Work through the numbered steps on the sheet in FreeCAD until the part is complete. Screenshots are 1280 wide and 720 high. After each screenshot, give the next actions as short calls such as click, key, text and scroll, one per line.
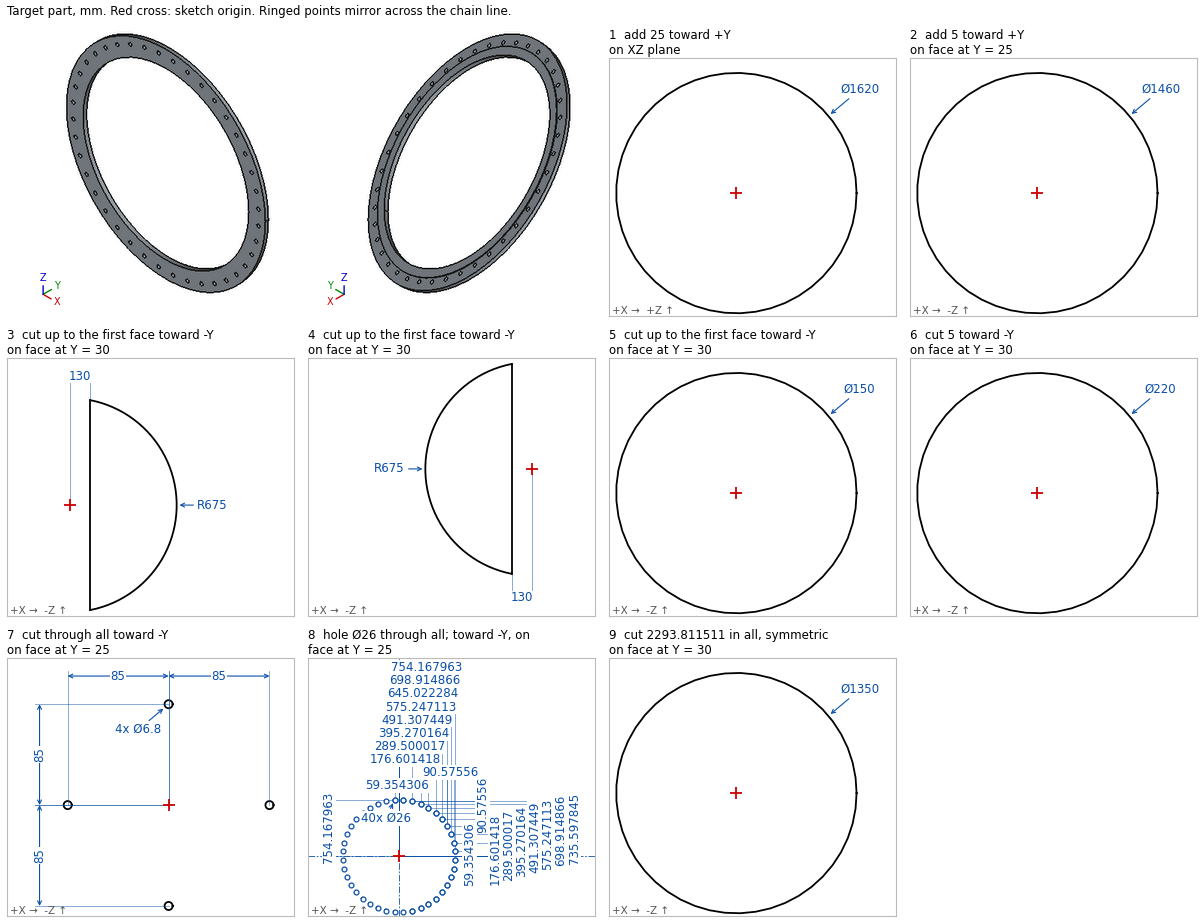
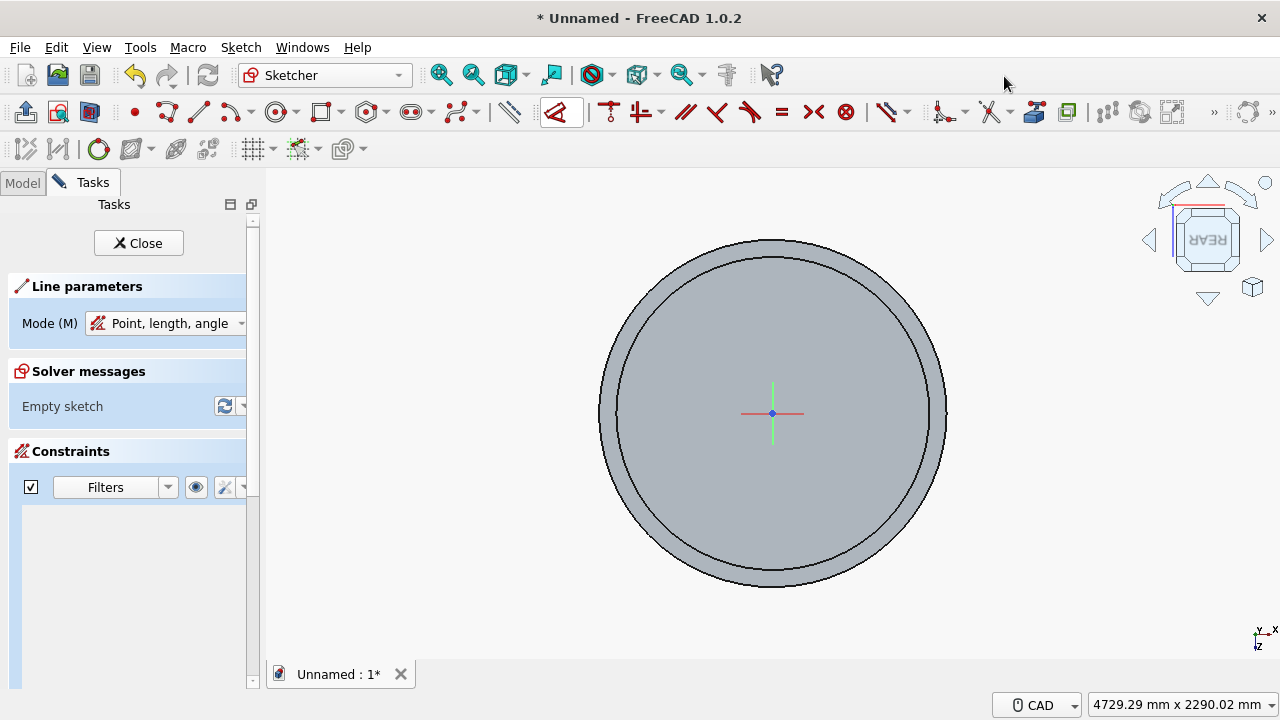
click(801, 271)
click(801, 556)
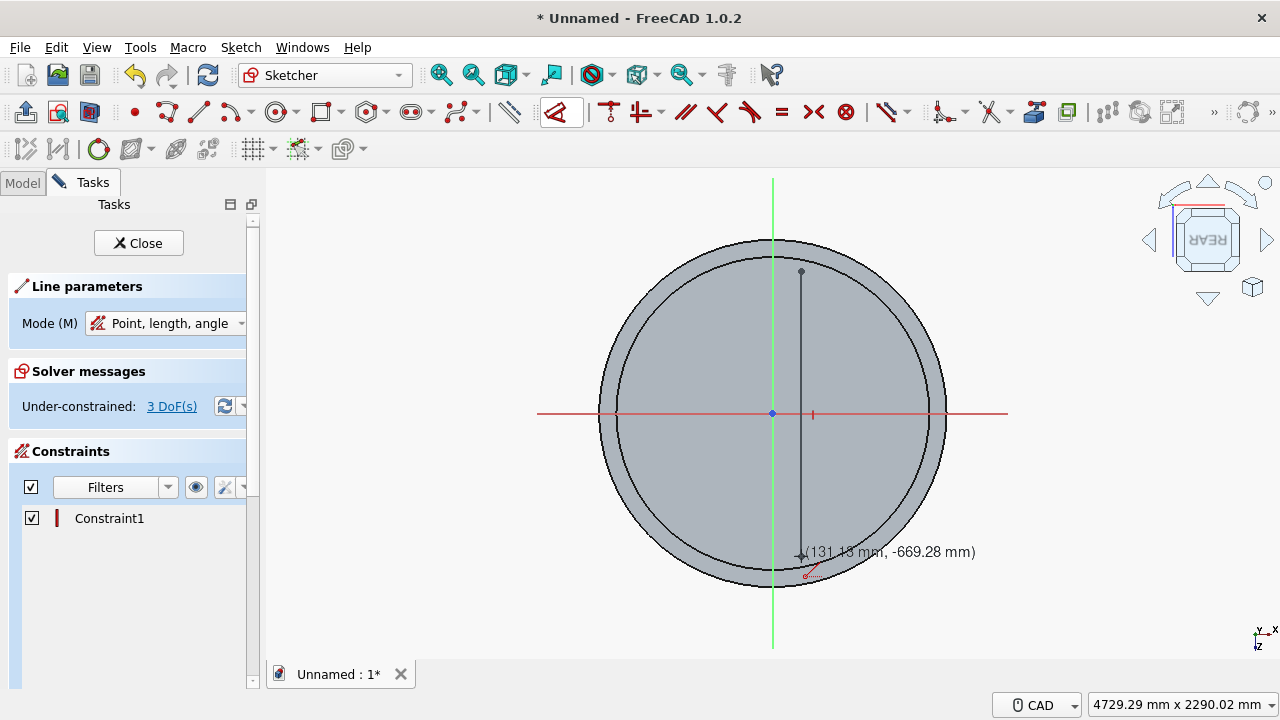
key(g)
key(3)
key(a)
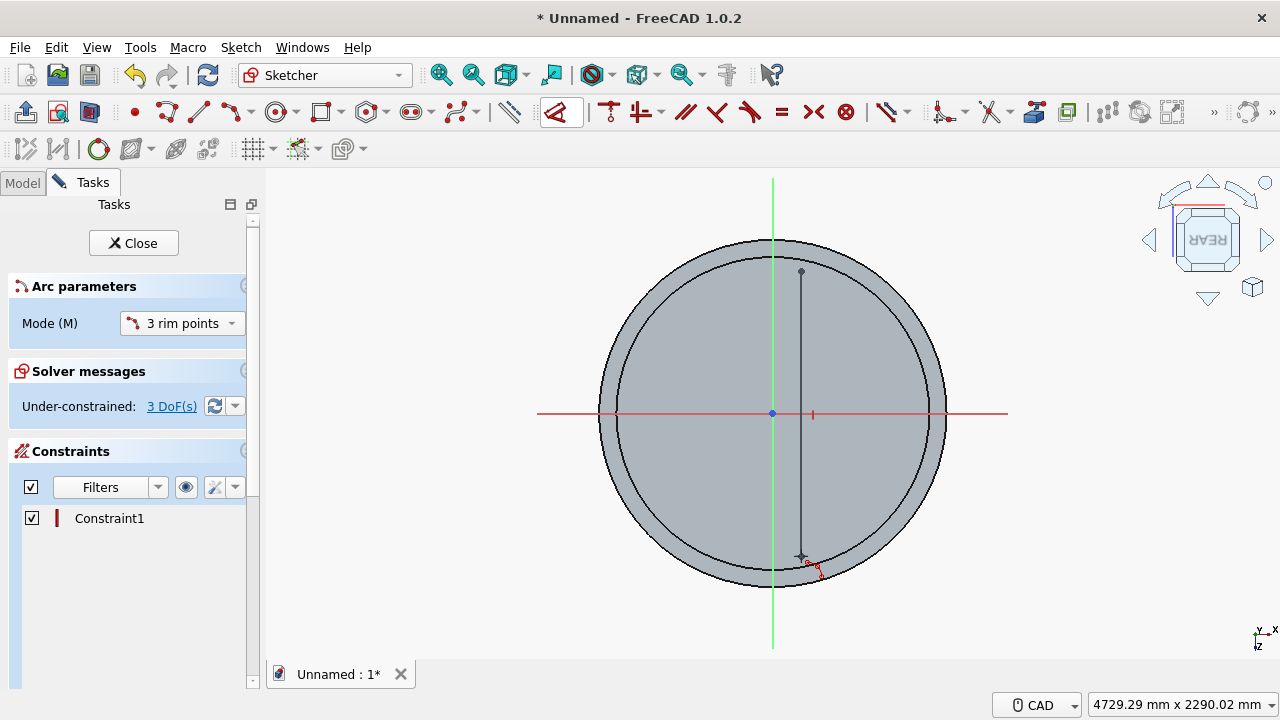
click(801, 557)
click(801, 272)
click(912, 453)
key(Escape)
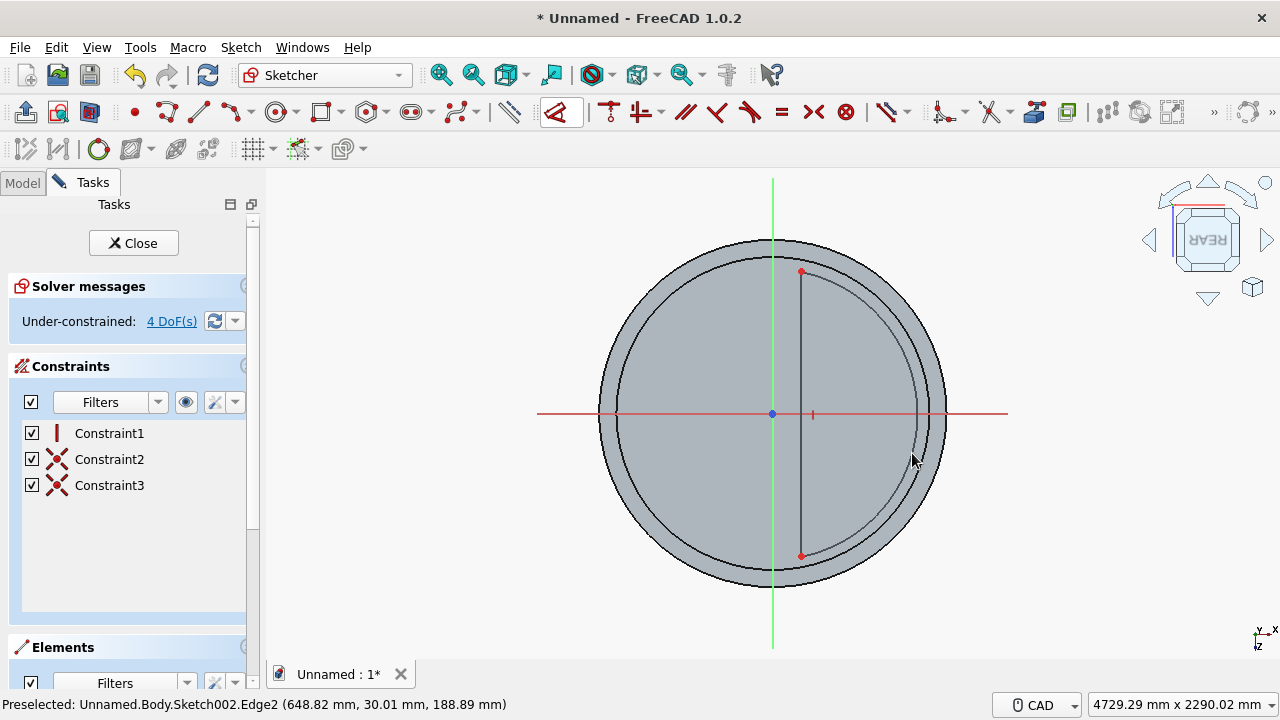
drag(762, 403, 783, 425)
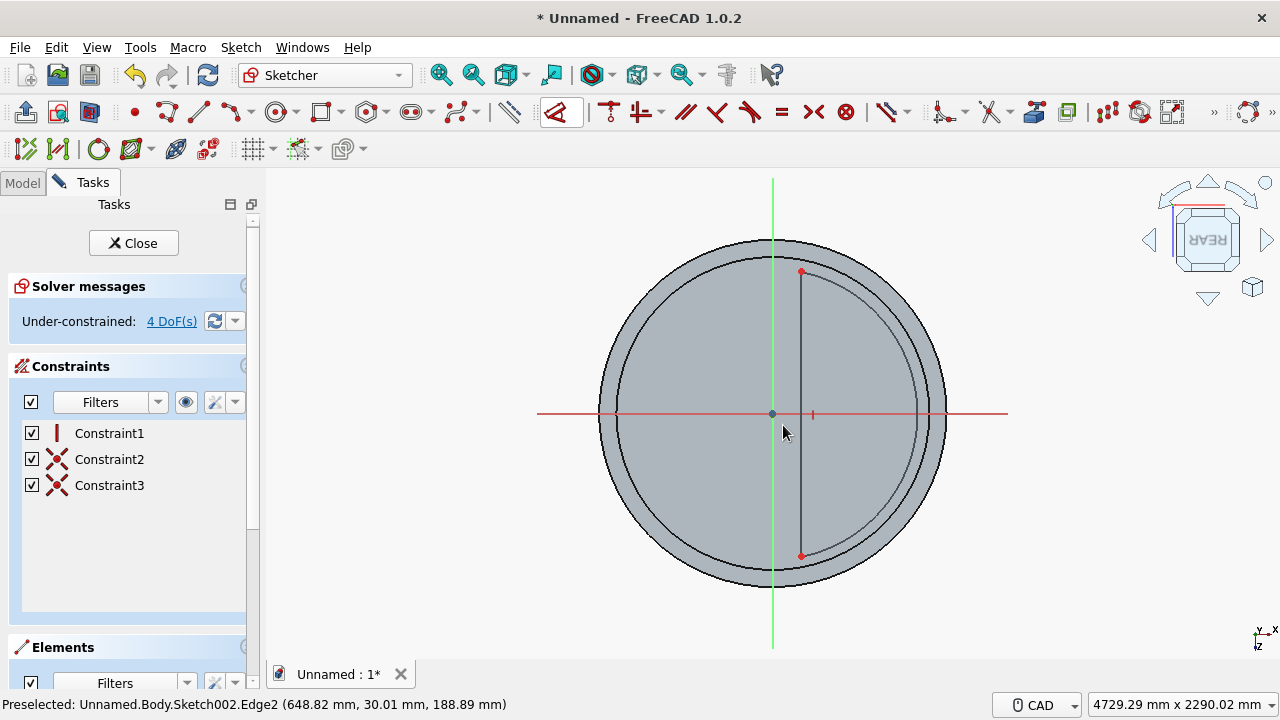
click(610, 112)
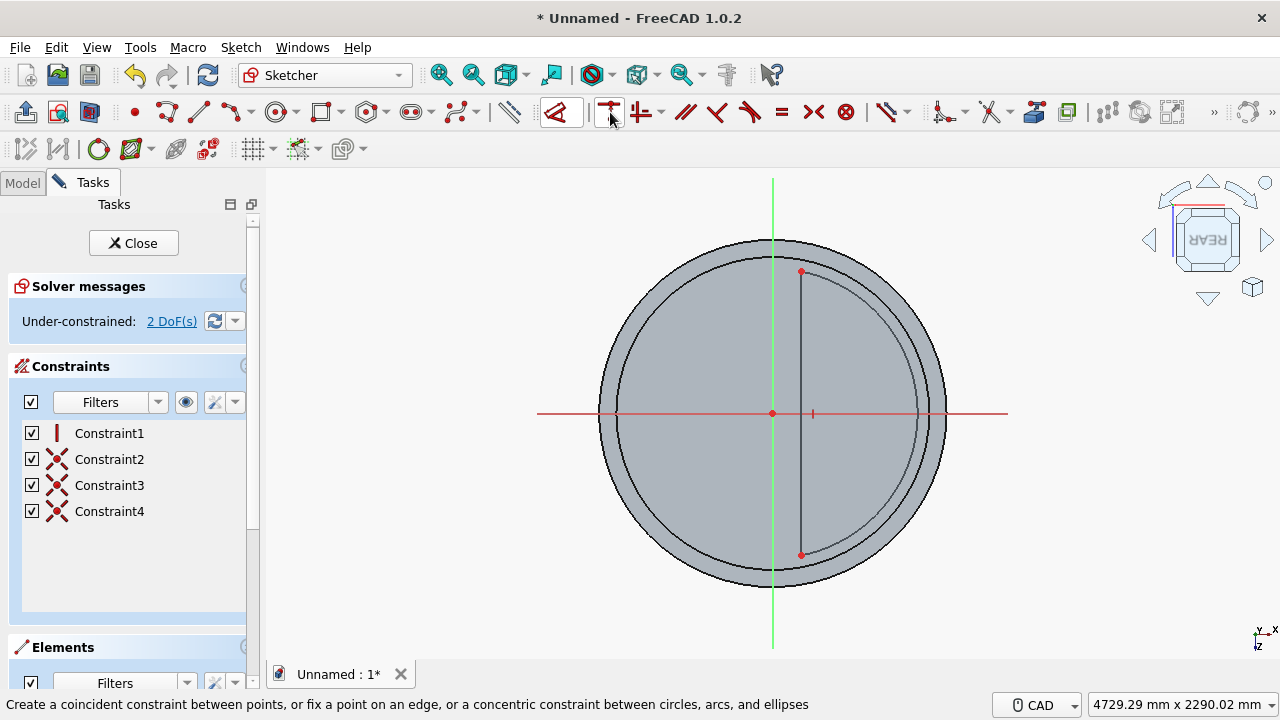
click(896, 489)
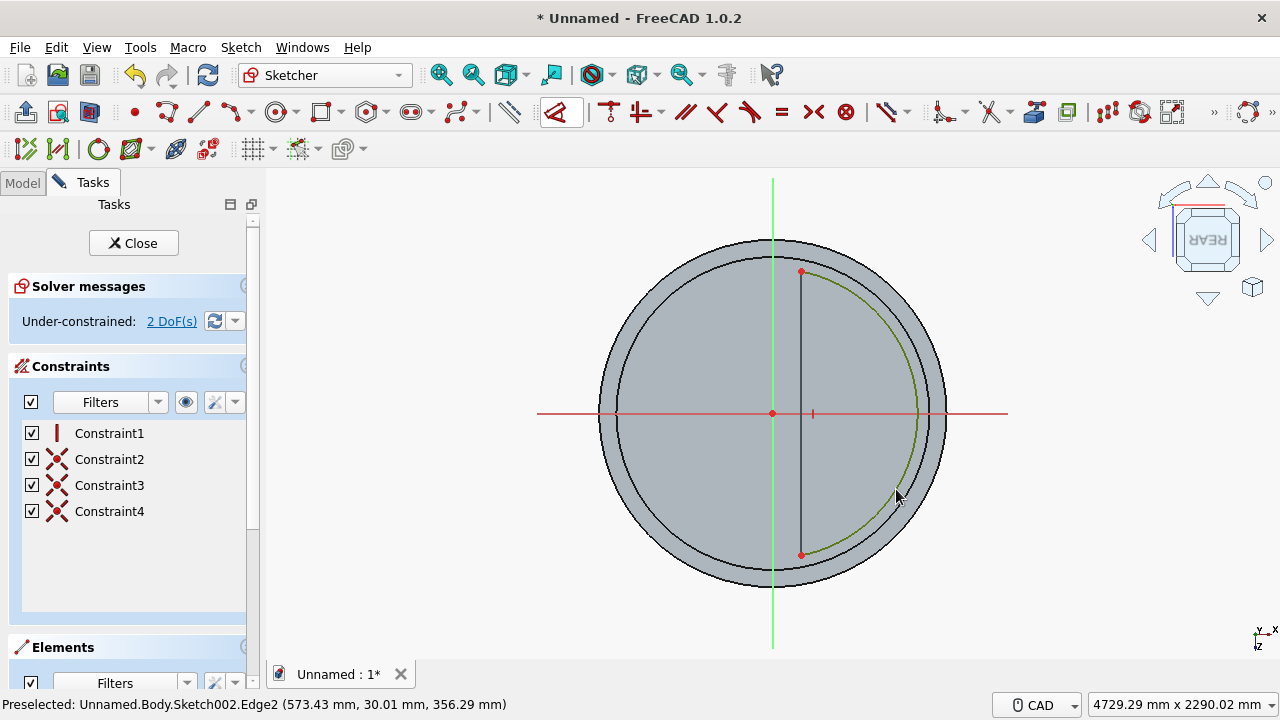
click(578, 112)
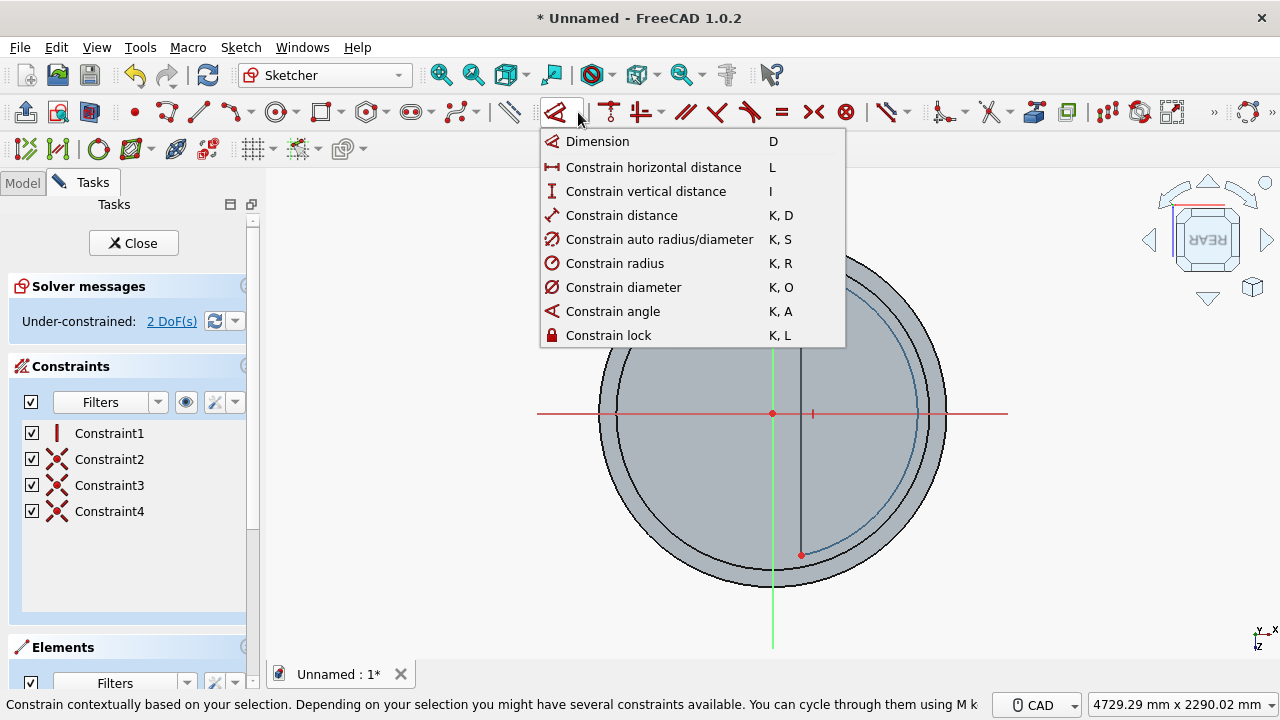
click(693, 263)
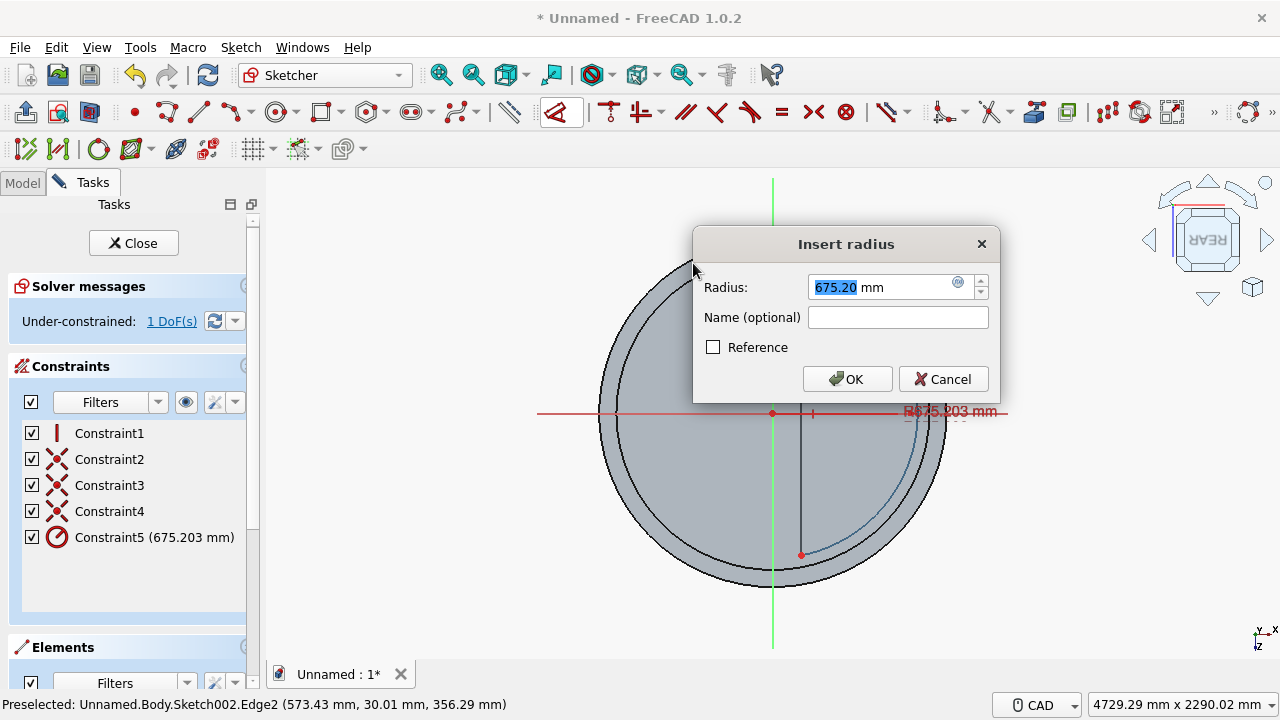
text(675)
key(Return)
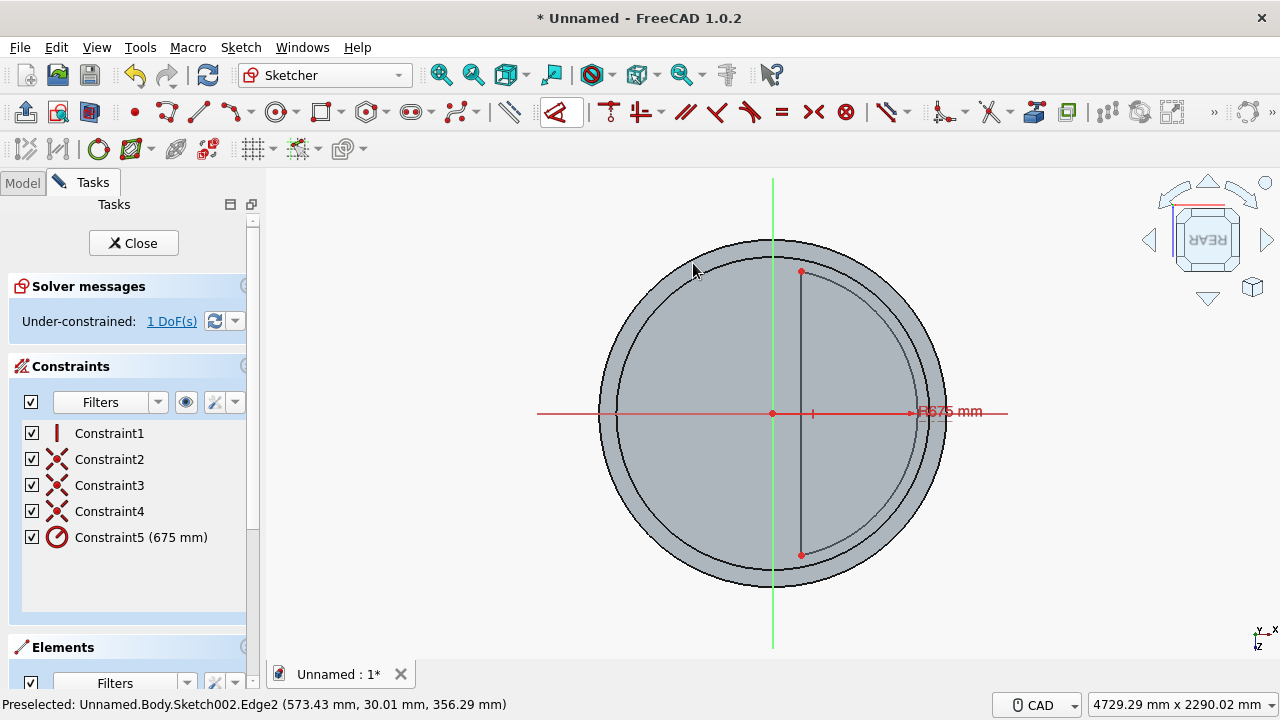
scroll(801, 272, up, 2)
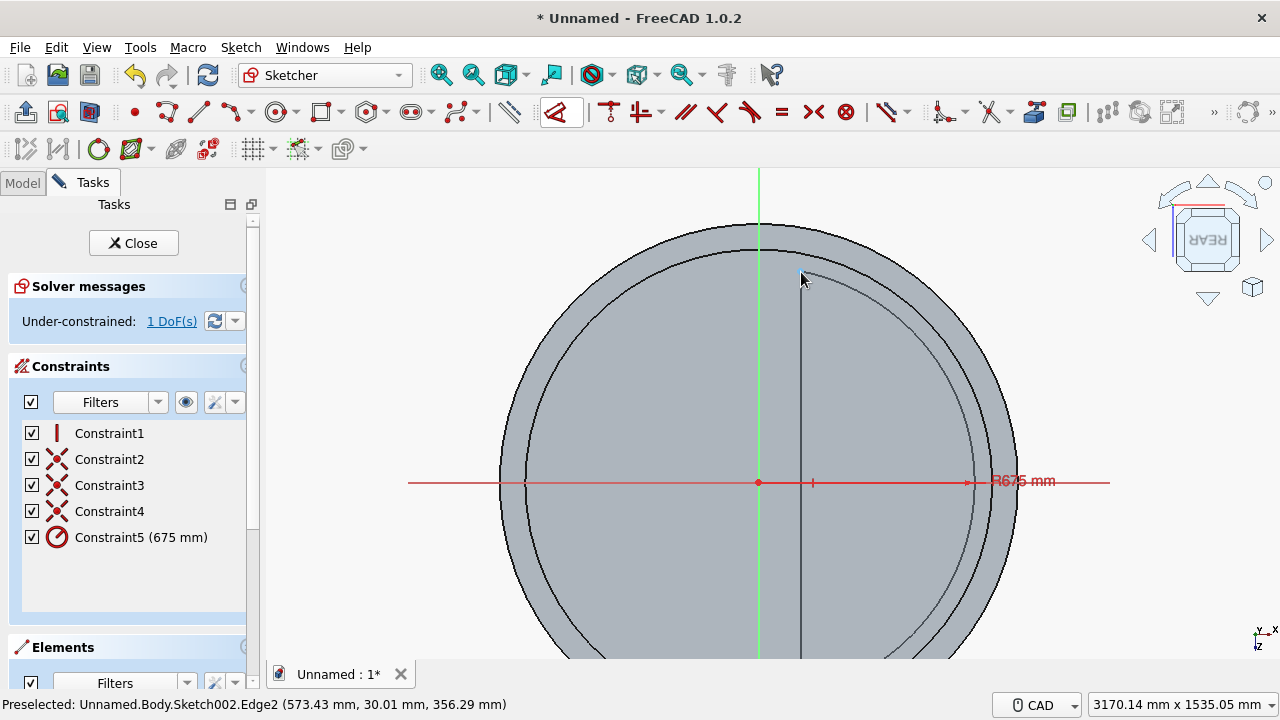
click(801, 271)